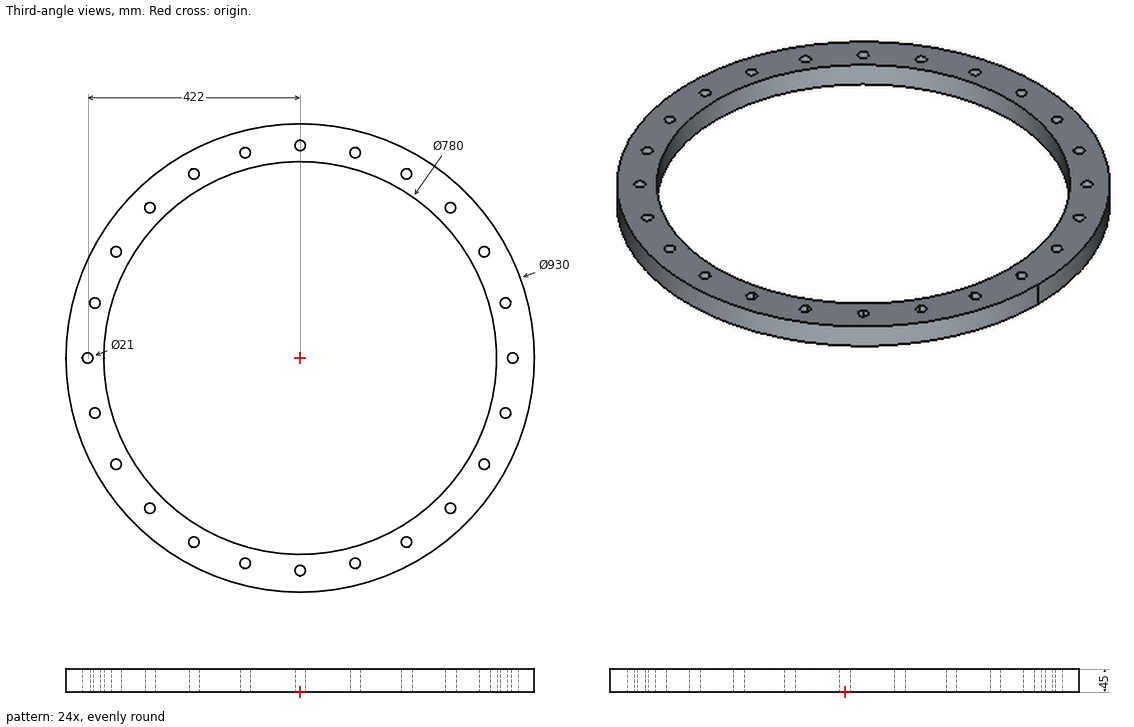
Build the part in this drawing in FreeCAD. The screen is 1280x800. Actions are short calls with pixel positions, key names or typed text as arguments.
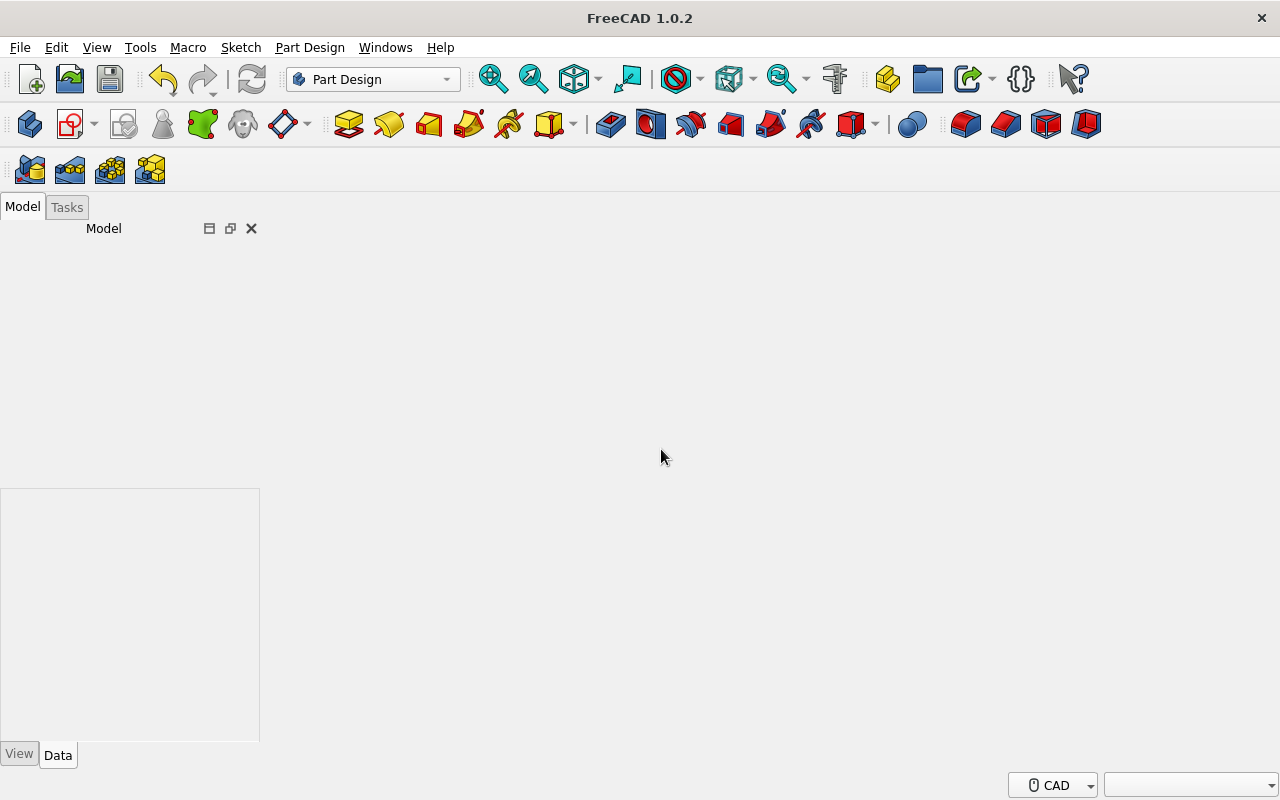
key(ctrl+n)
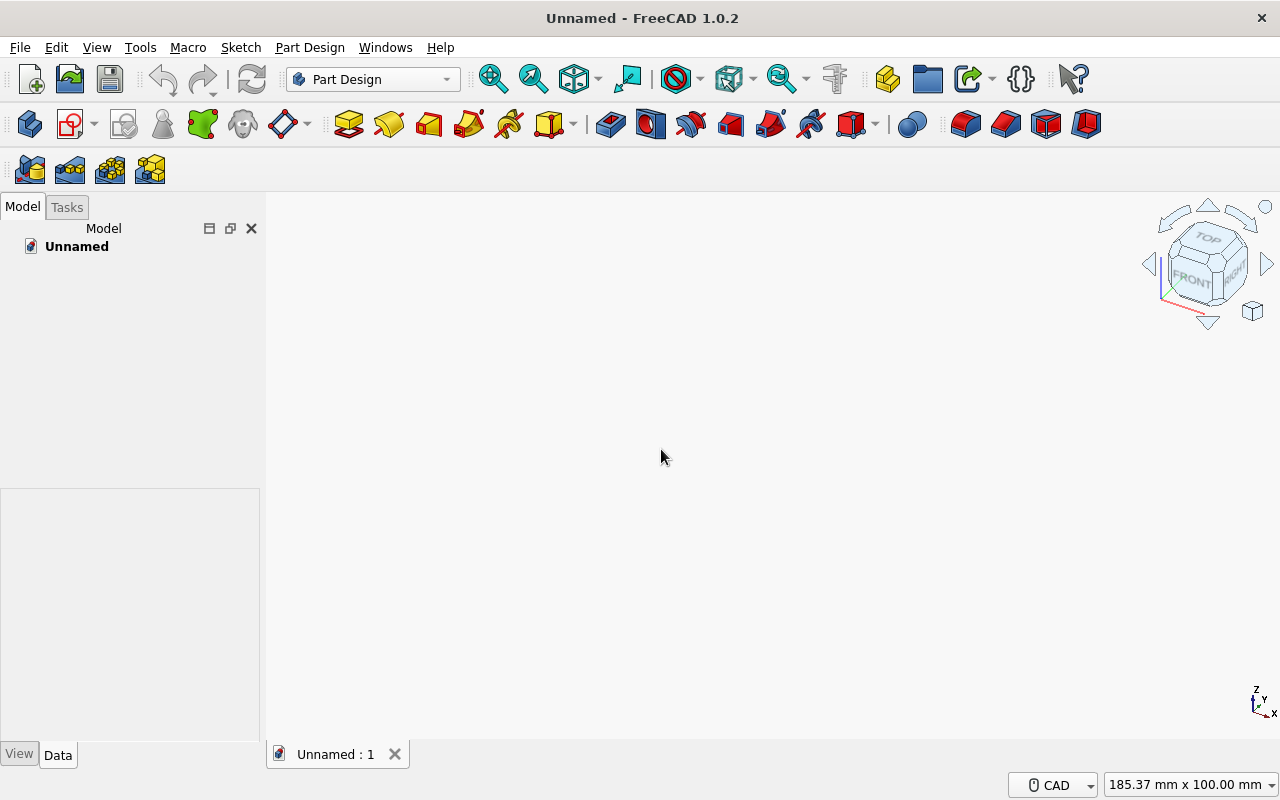
click(70, 124)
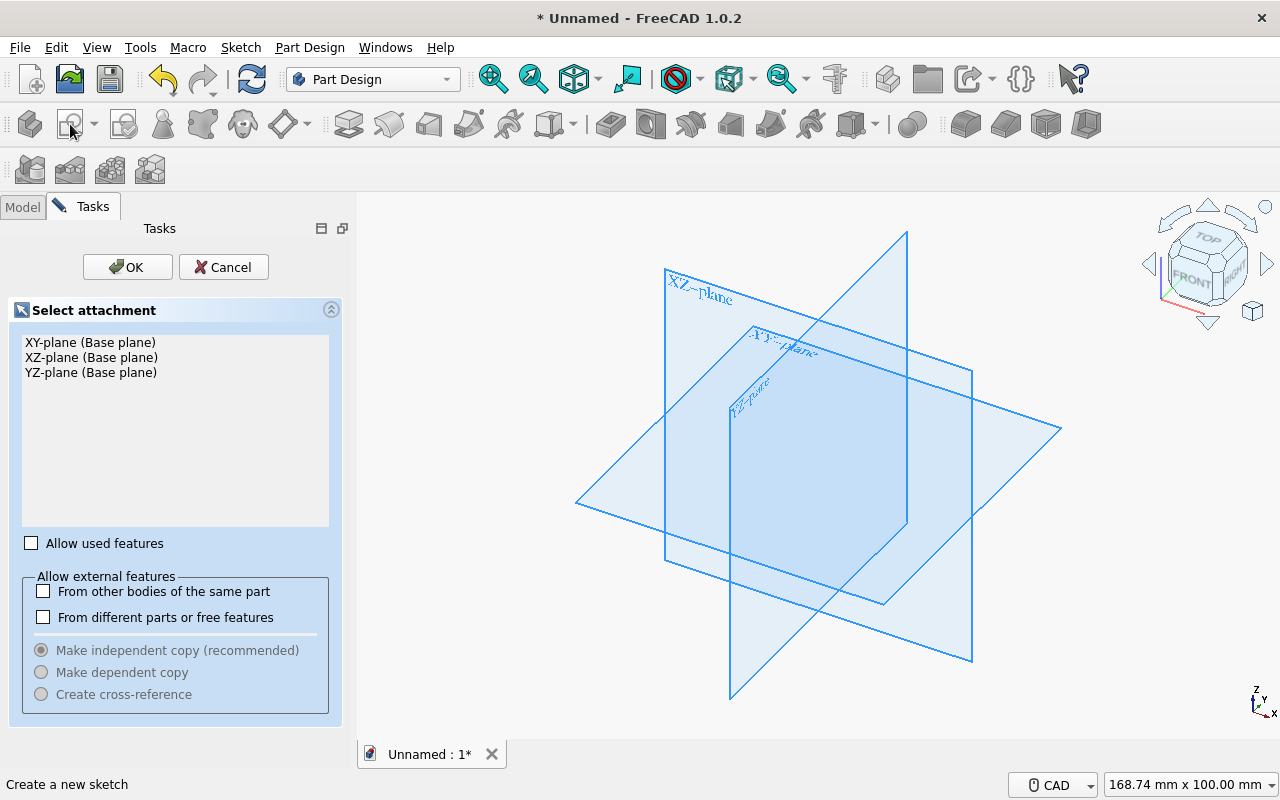
click(82, 342)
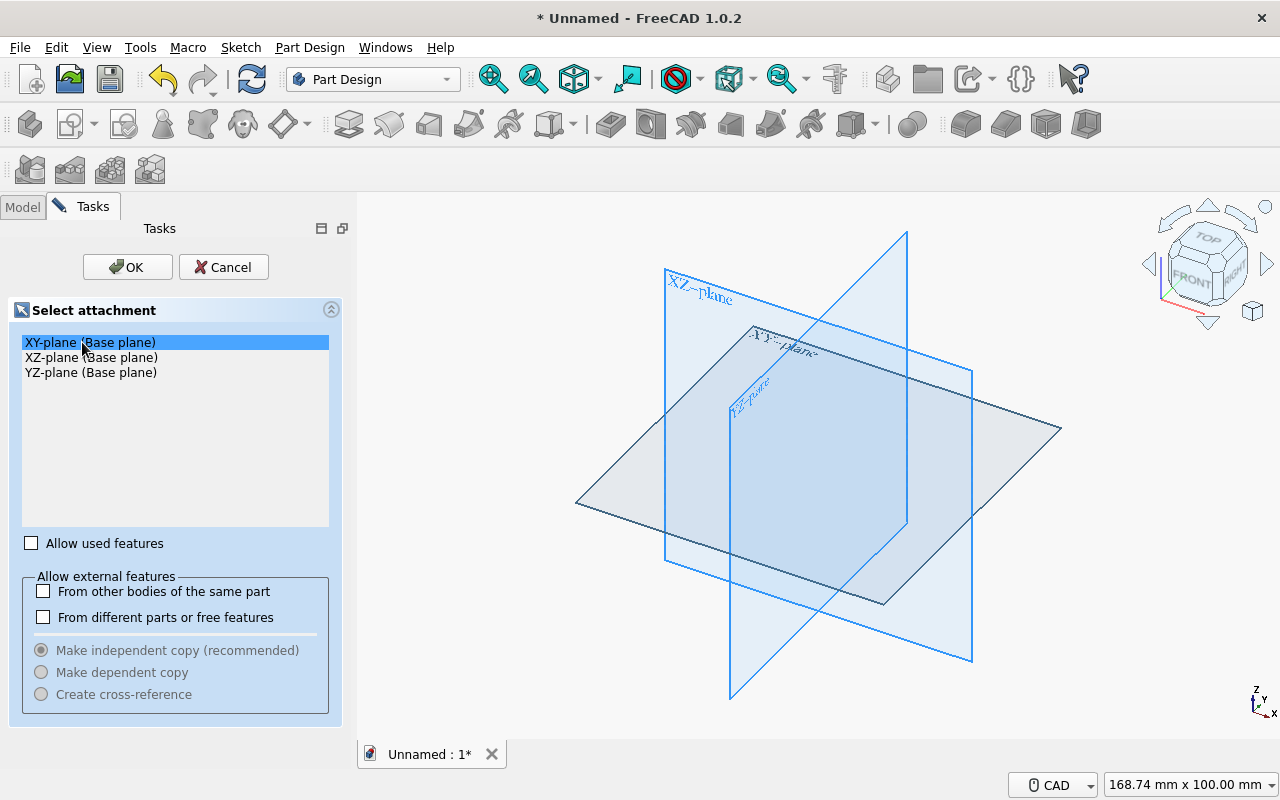
click(128, 267)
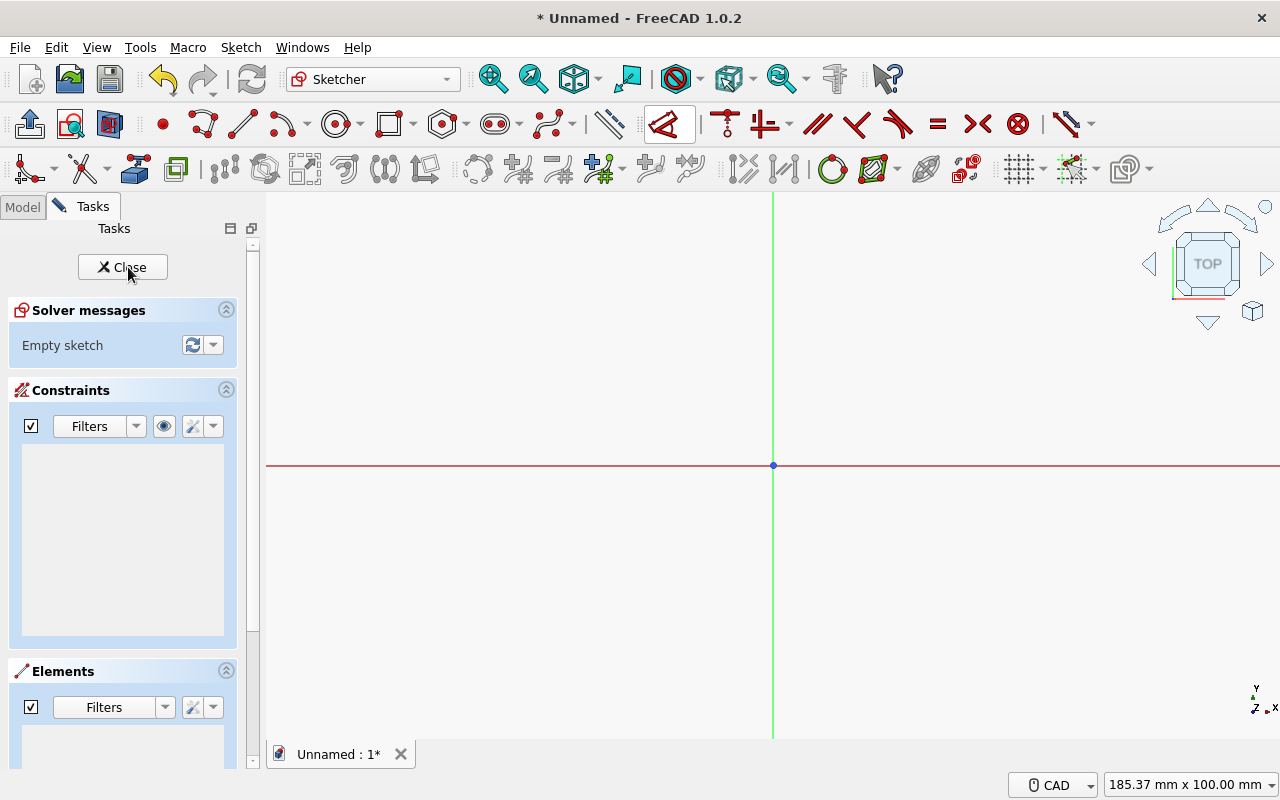
scroll(699, 466, down, 13)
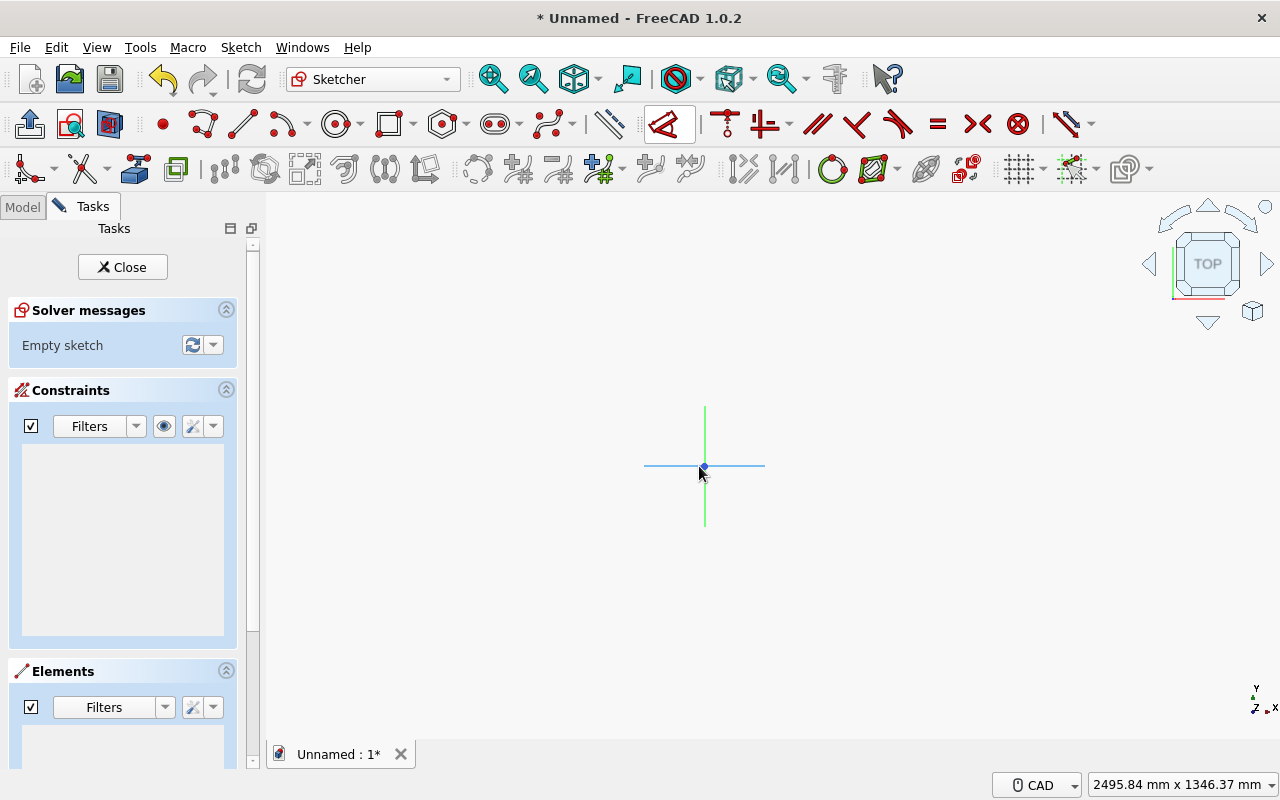
click(336, 124)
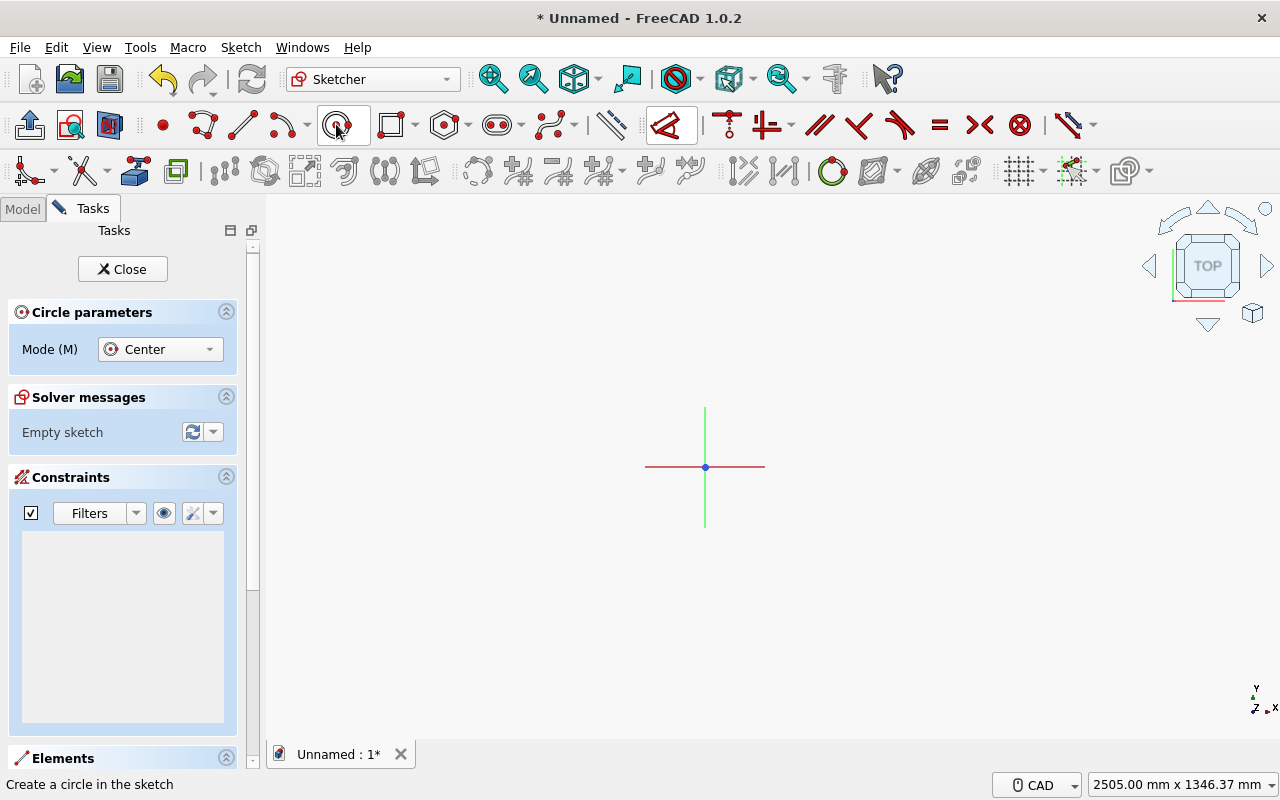
click(705, 467)
click(838, 334)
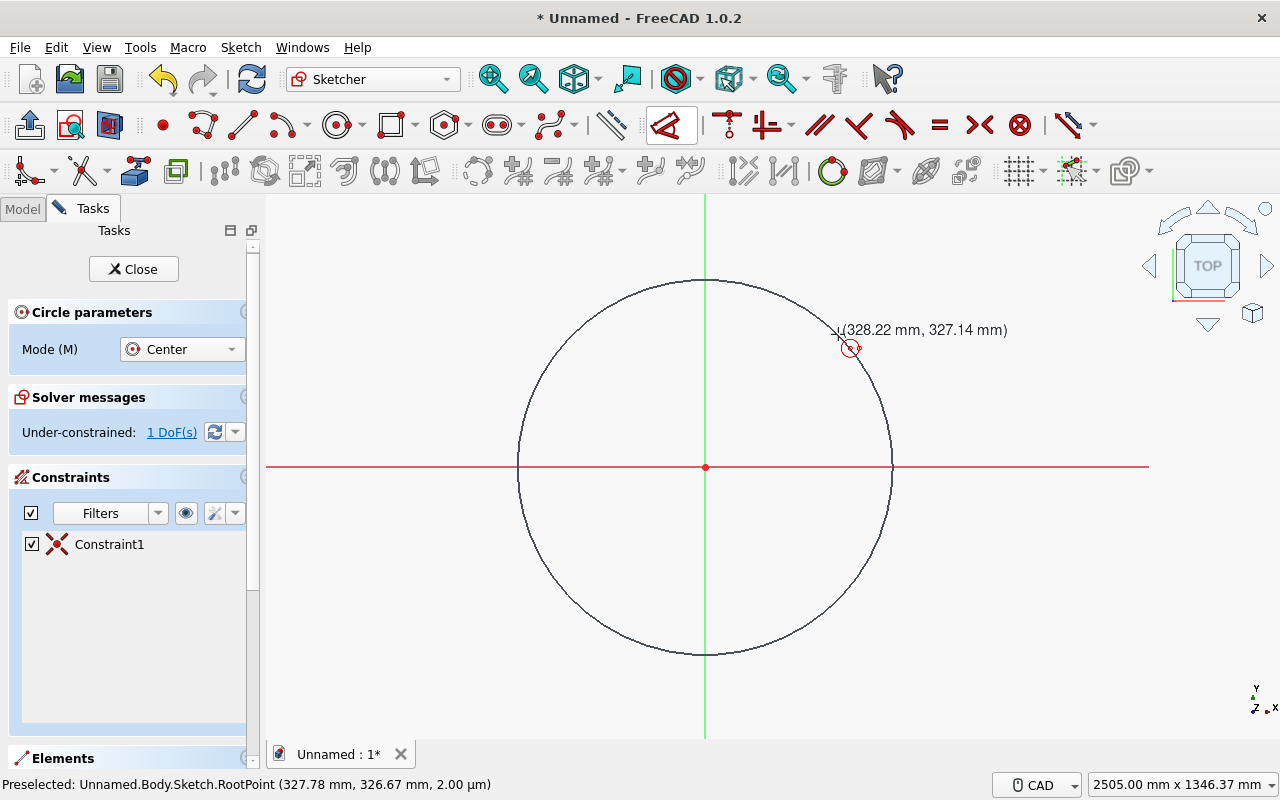
click(705, 467)
click(817, 356)
key(Escape)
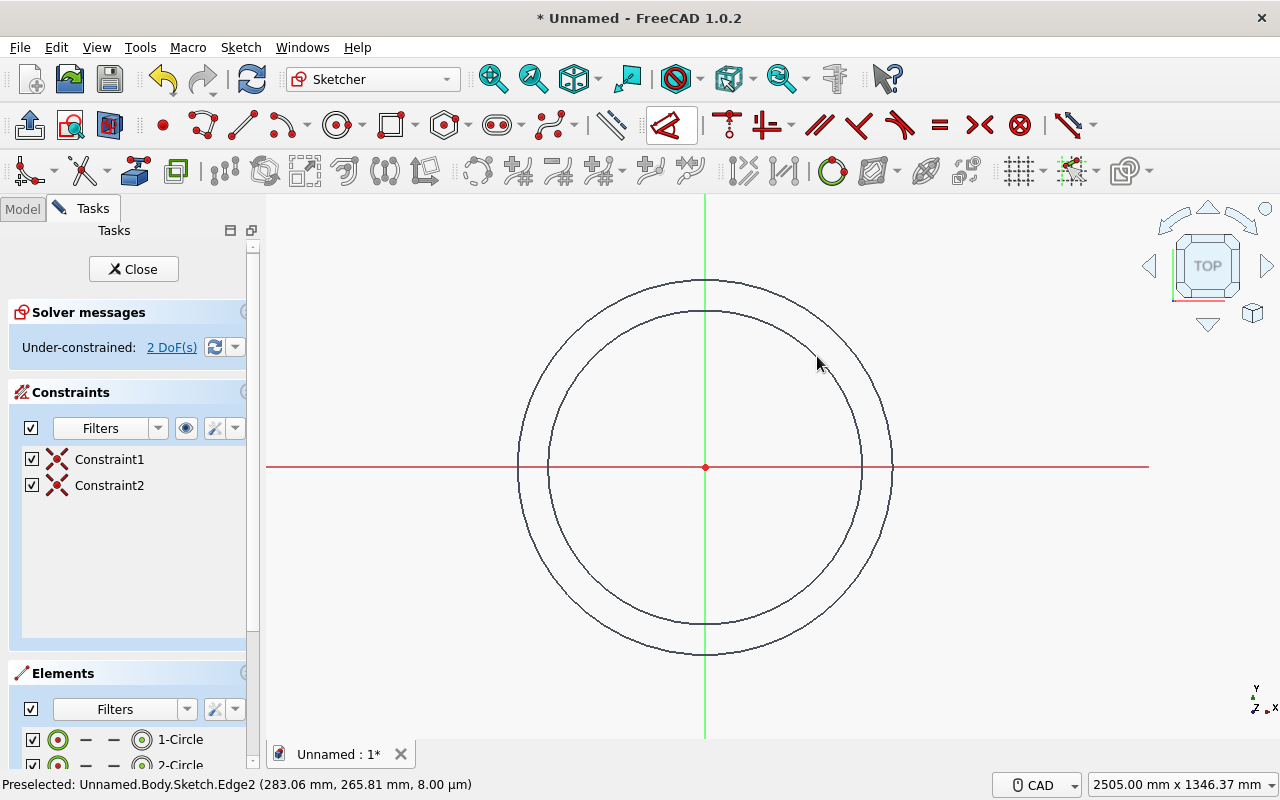
key(d)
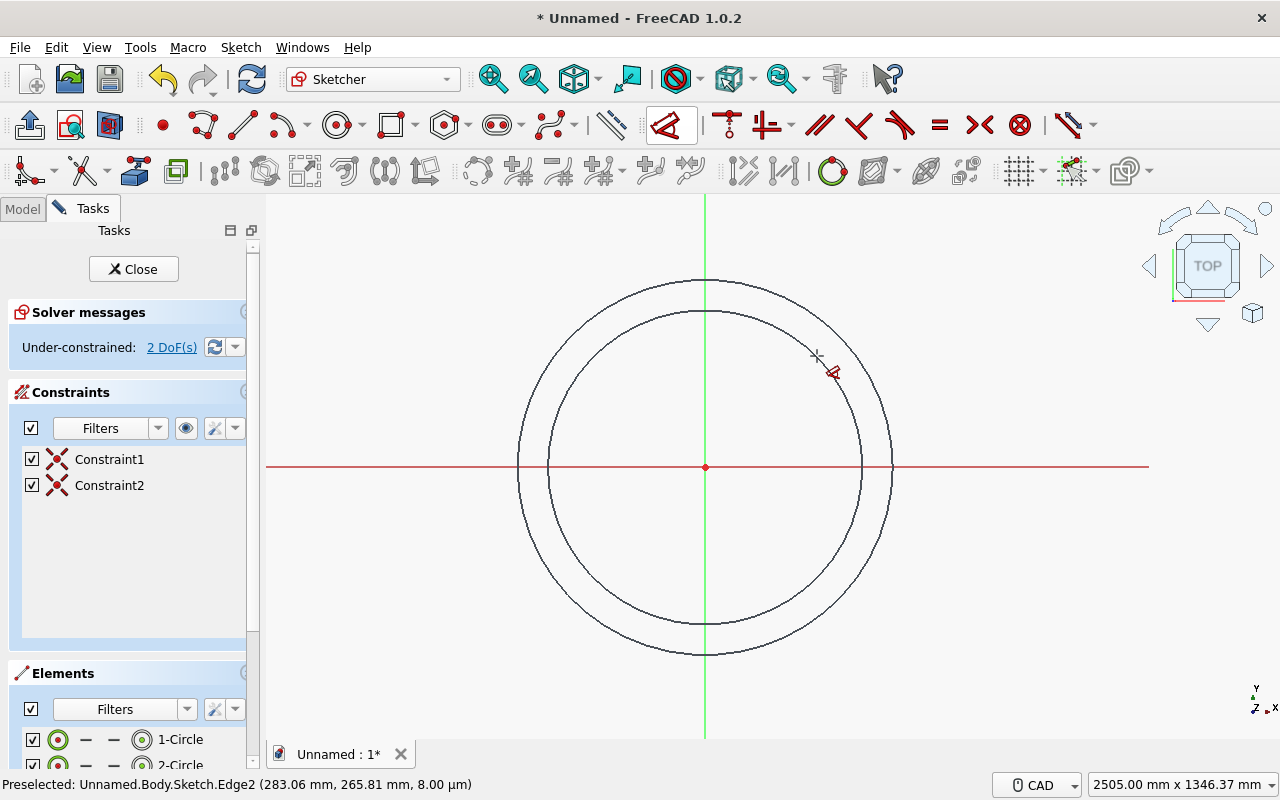
click(837, 334)
click(859, 311)